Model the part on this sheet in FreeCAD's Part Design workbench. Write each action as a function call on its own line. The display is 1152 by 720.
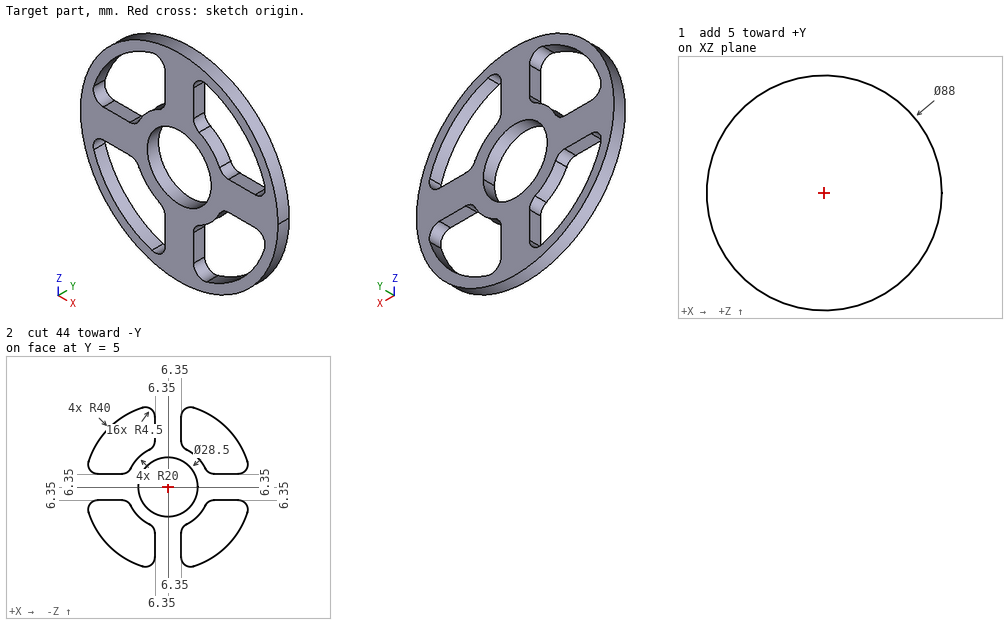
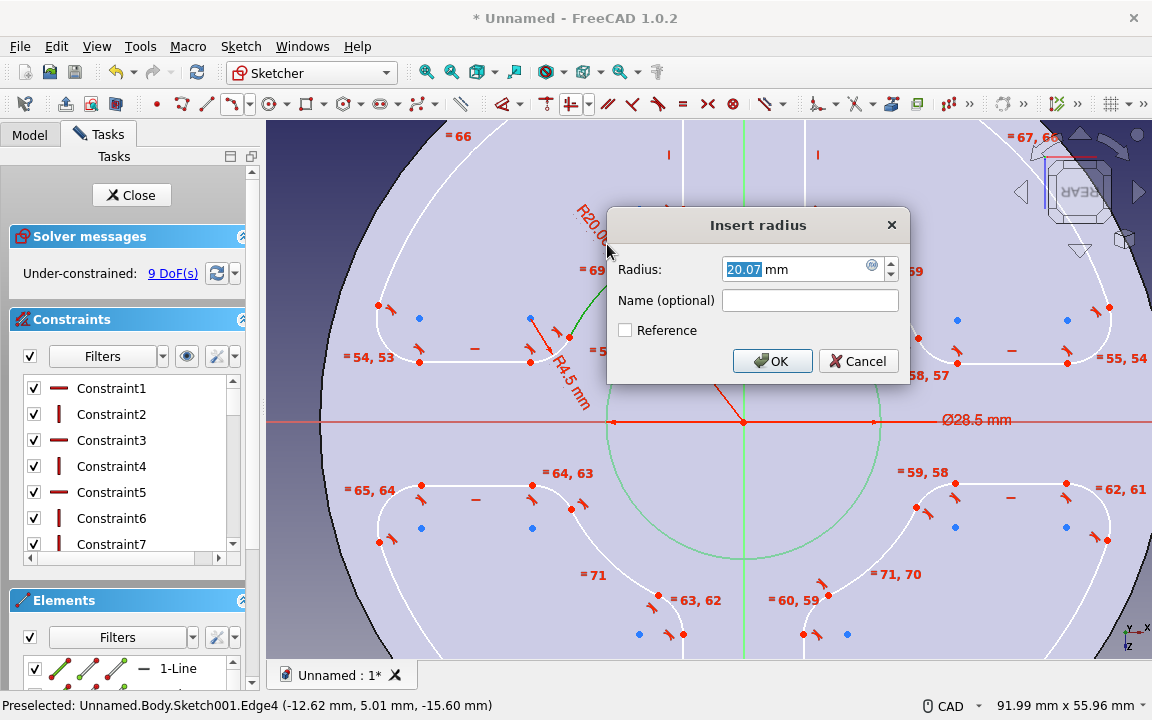
text(20)
key(Return)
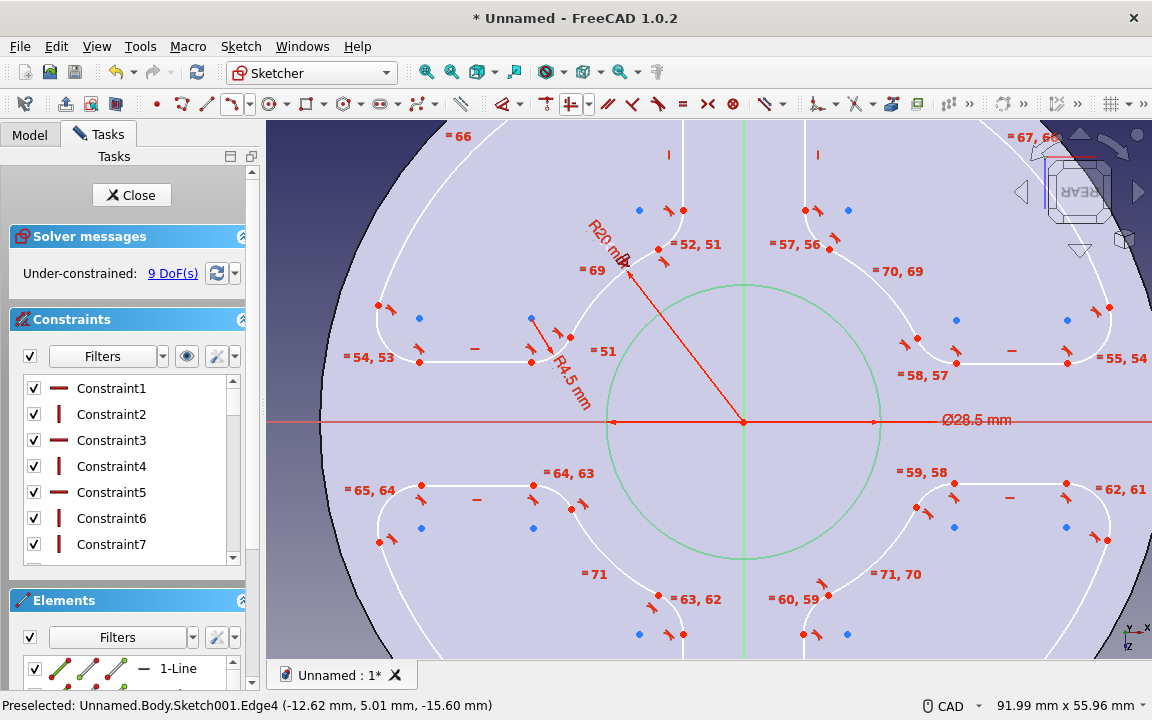
click(426, 208)
click(399, 190)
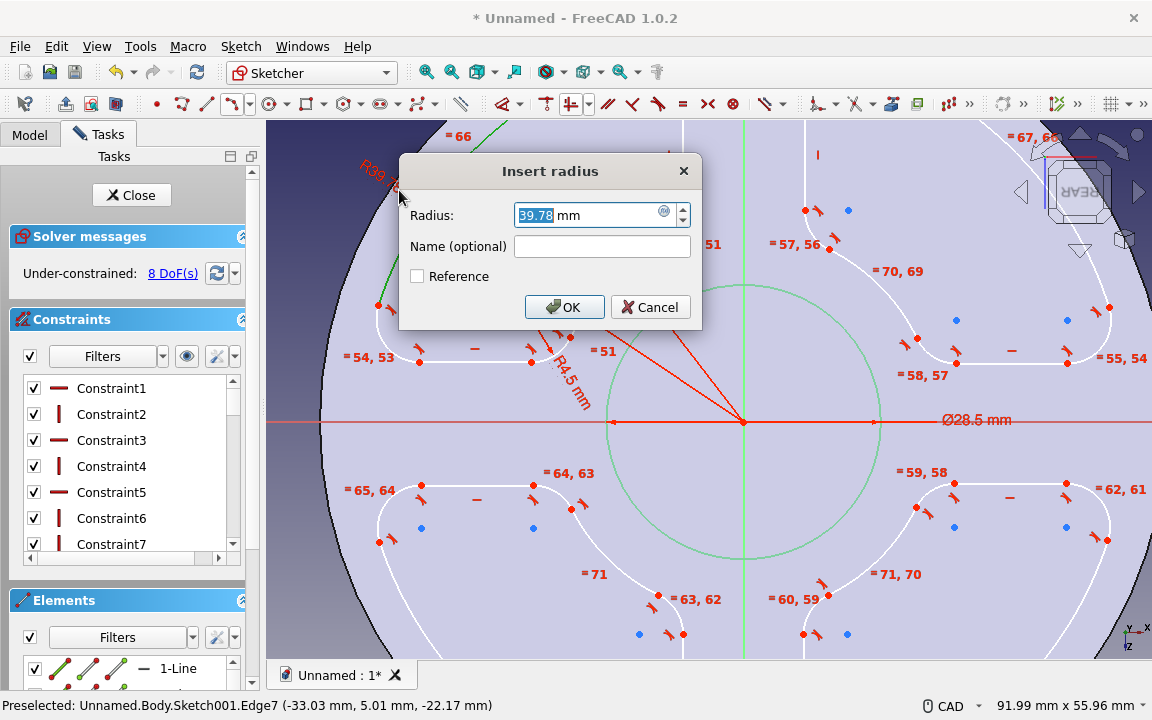
text(40)
key(Return)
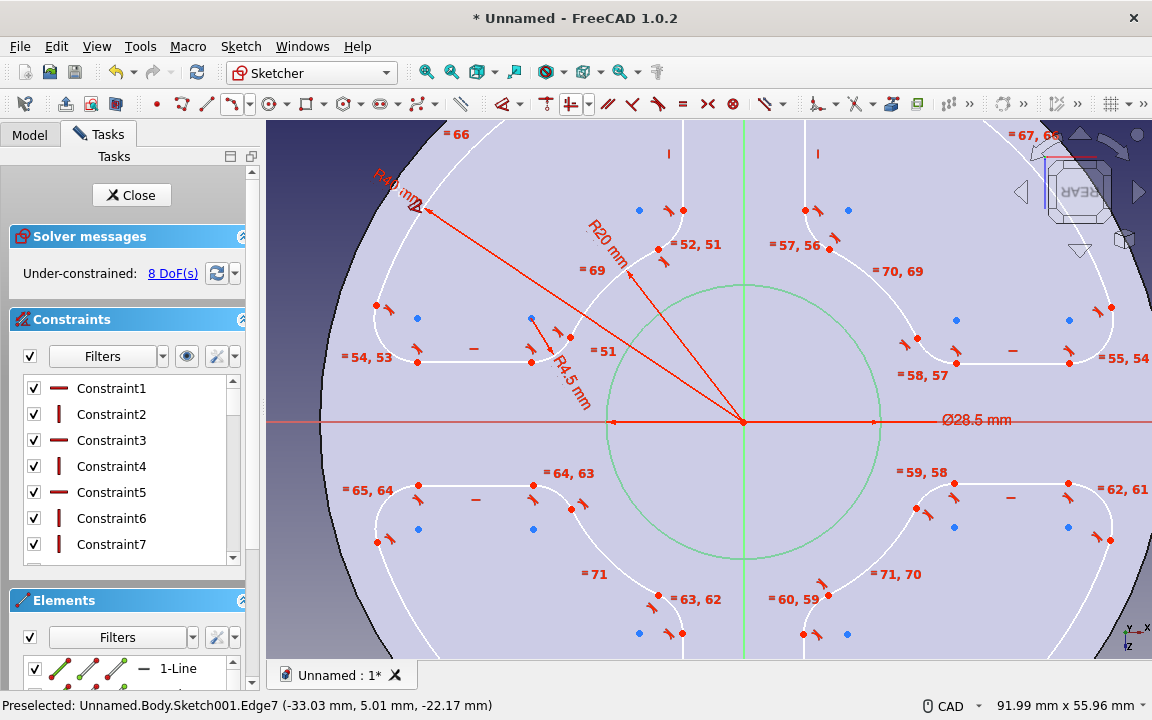
click(418, 362)
click(384, 392)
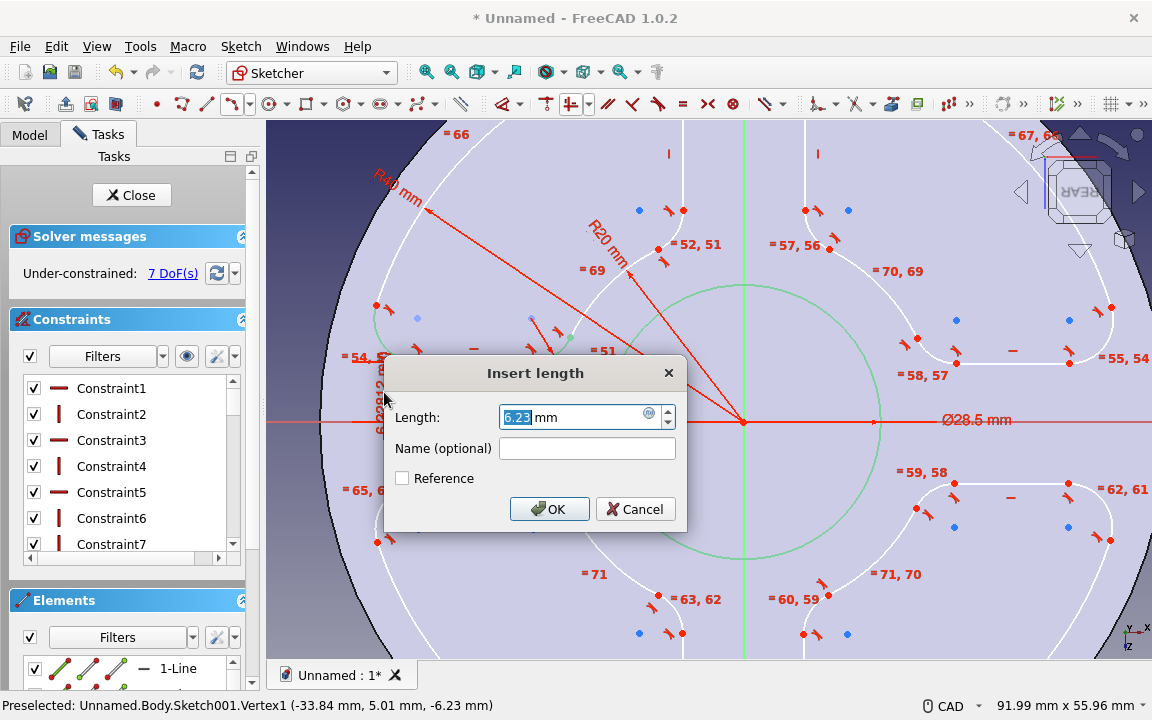
text(6.35)
key(Return)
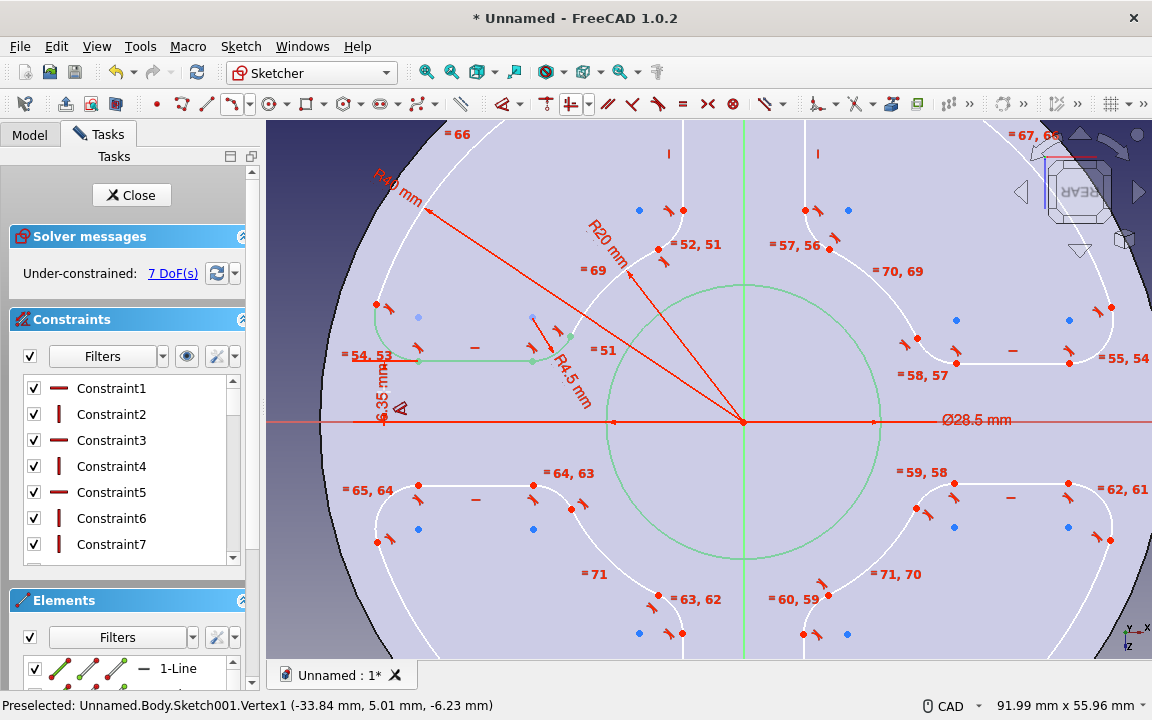
click(683, 210)
click(713, 176)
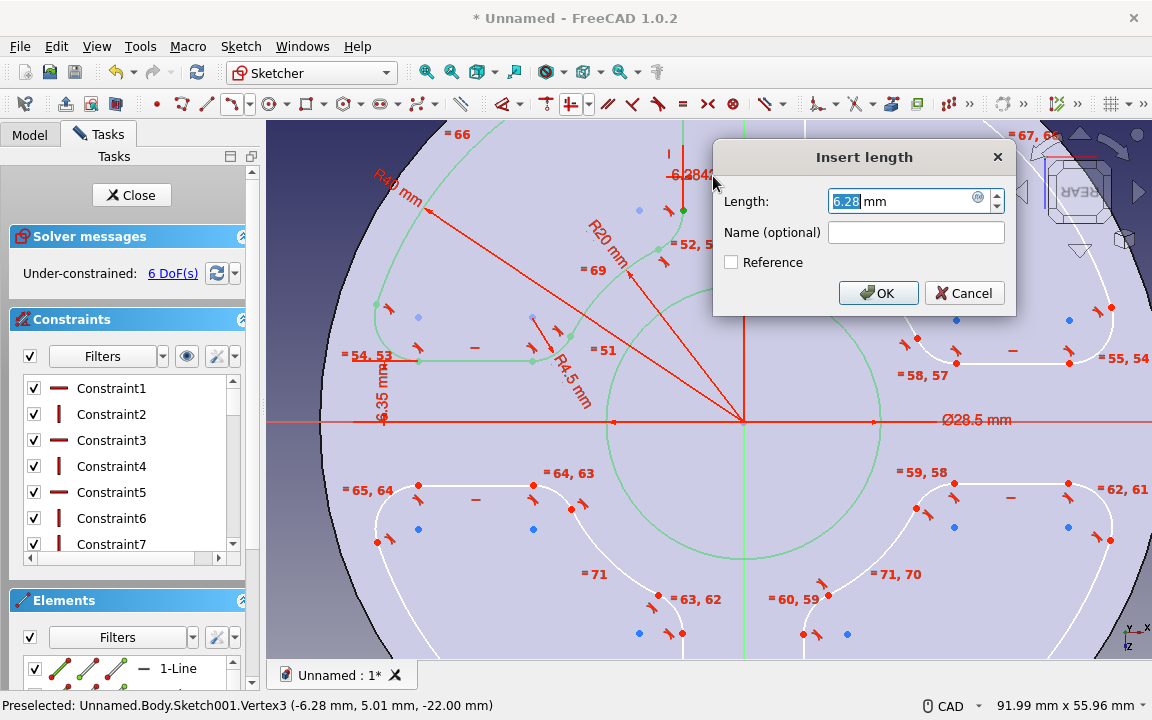
text(6.35)
key(Return)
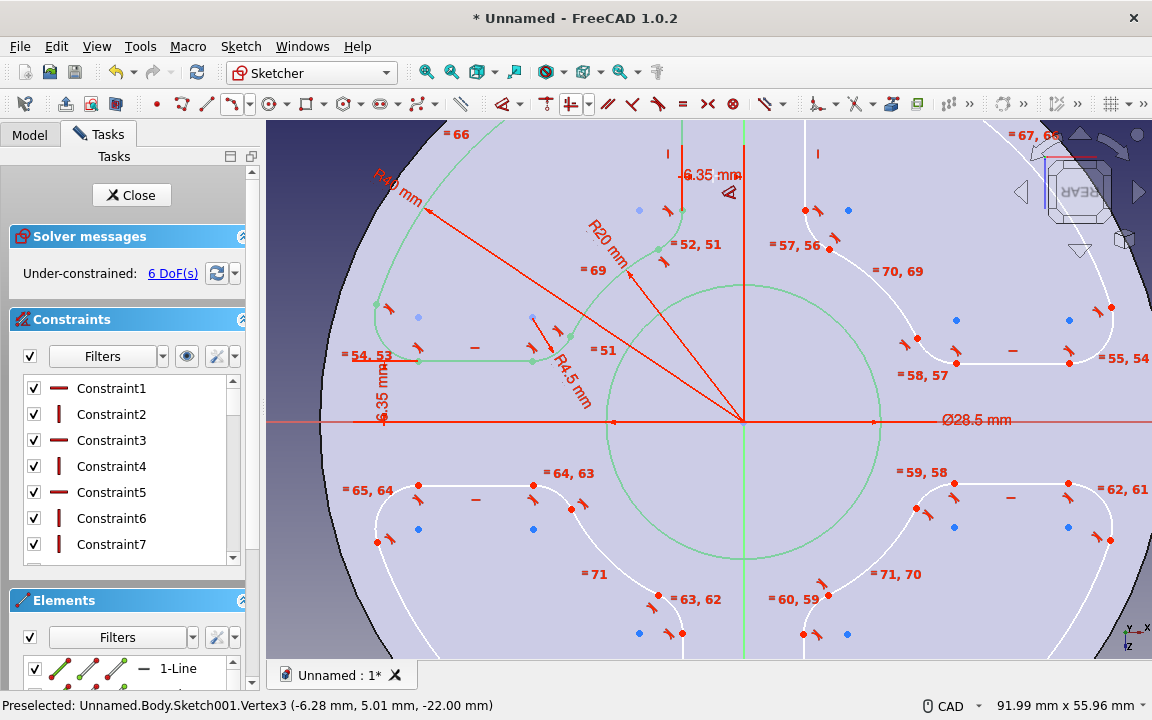
click(956, 364)
click(710, 393)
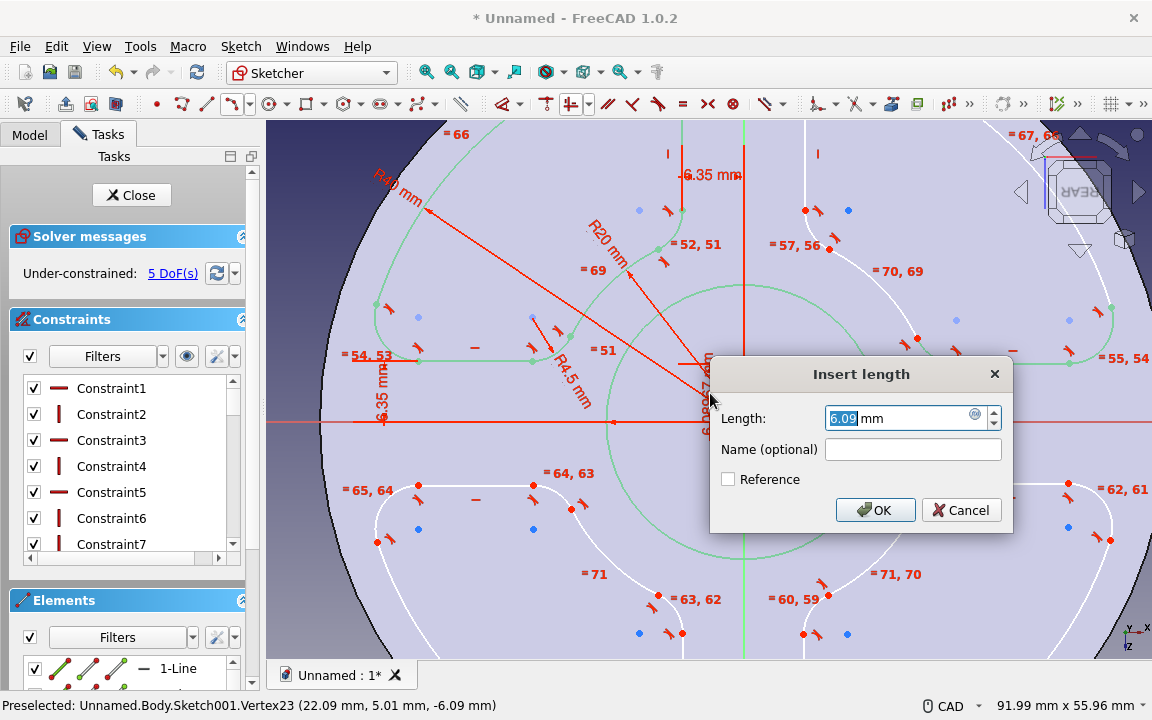
text(6.35)
key(Return)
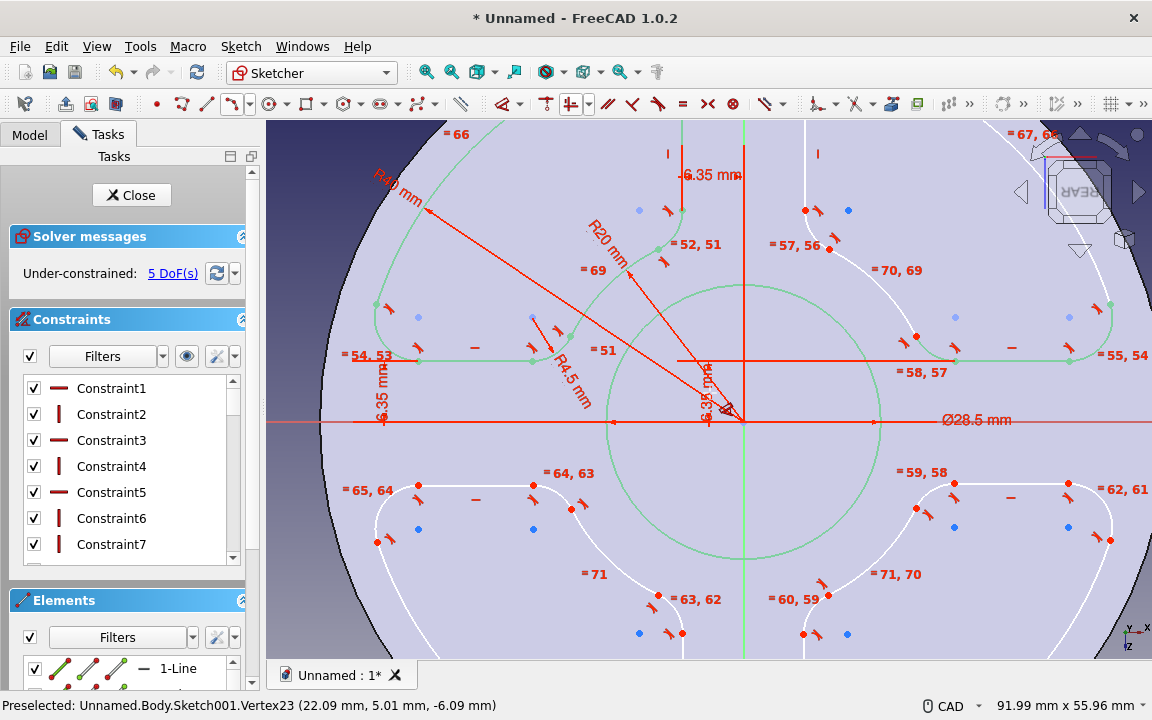
scroll(556, 363, down, 4)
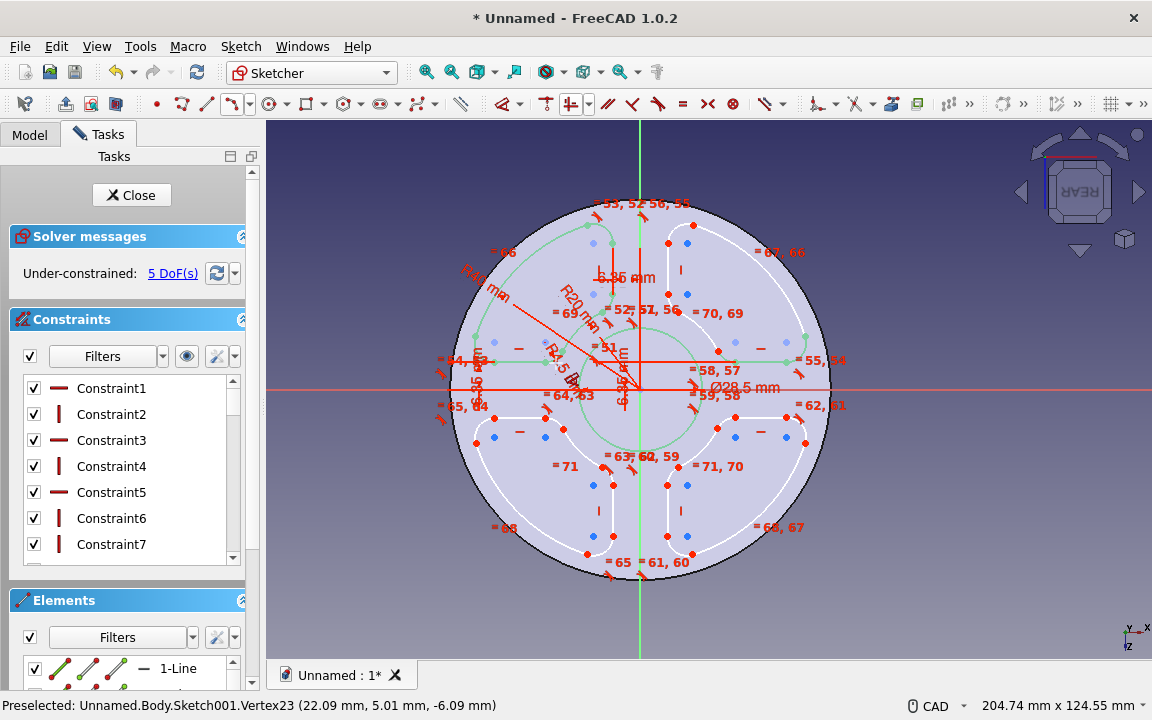
scroll(668, 244, up, 2)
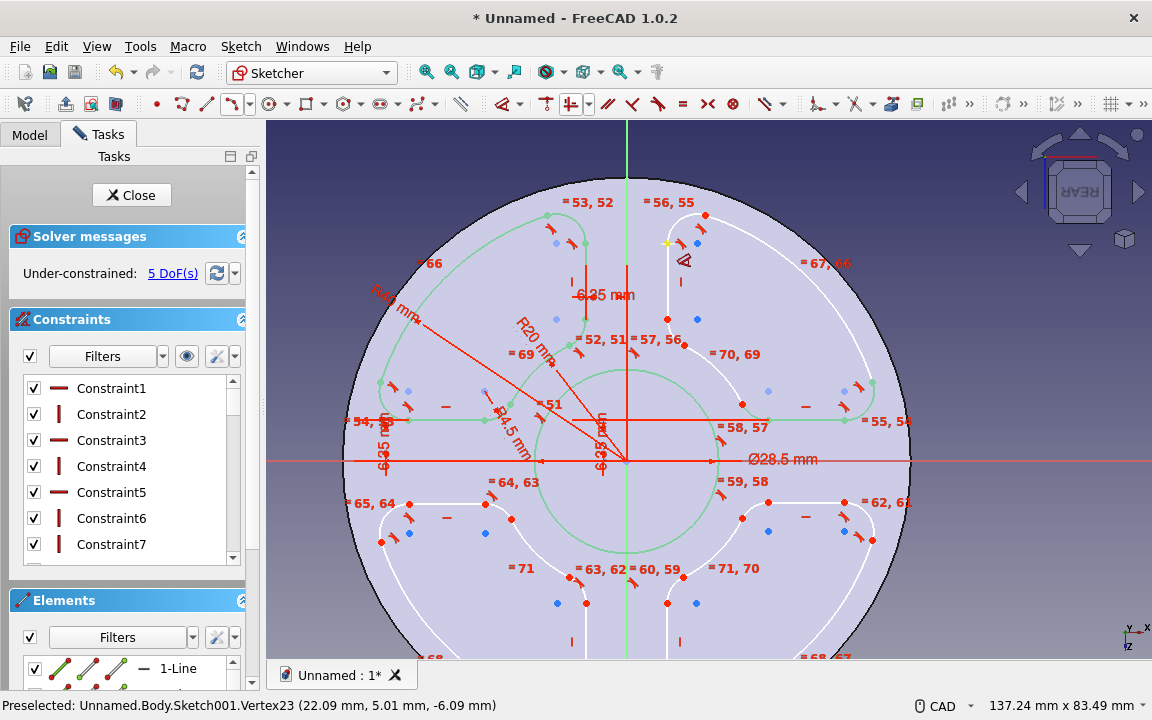
click(668, 243)
click(647, 209)